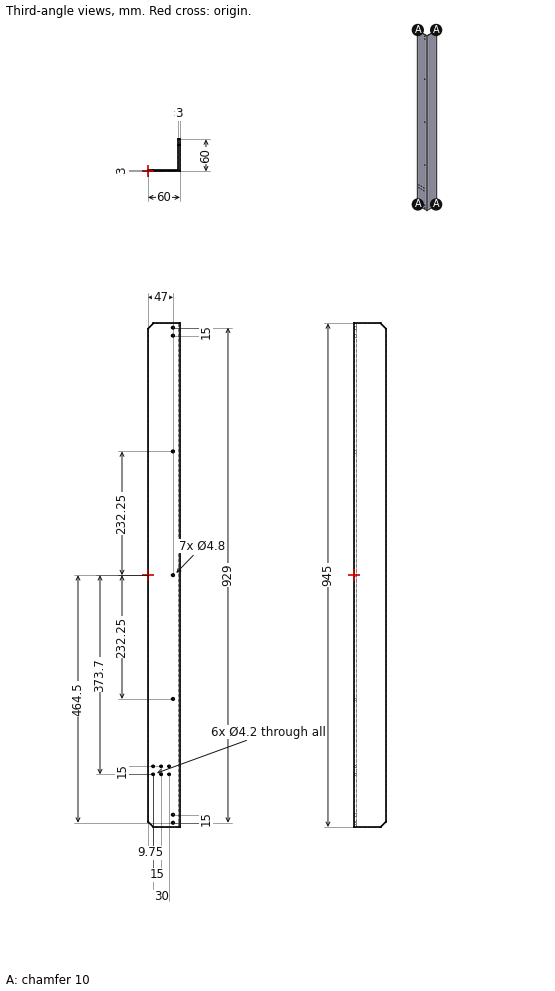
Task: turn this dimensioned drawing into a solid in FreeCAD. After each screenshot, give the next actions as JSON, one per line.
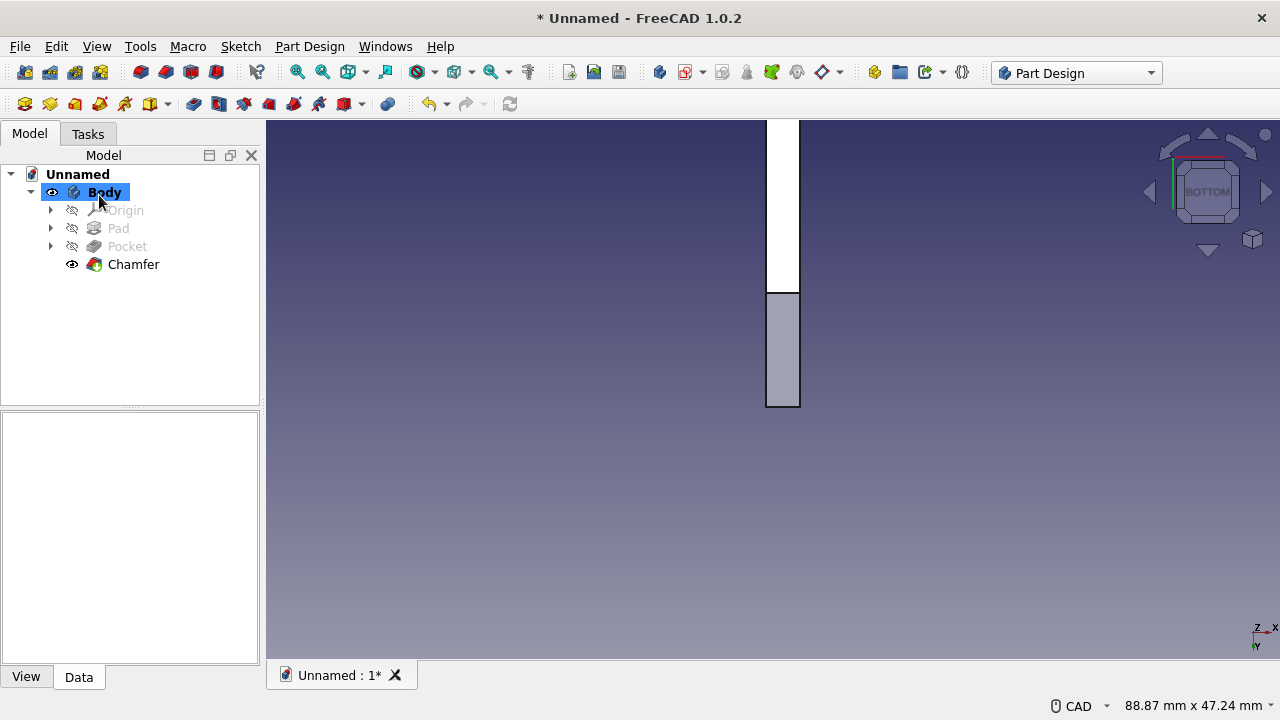
{"action": "left_click", "coordinate": [298, 72]}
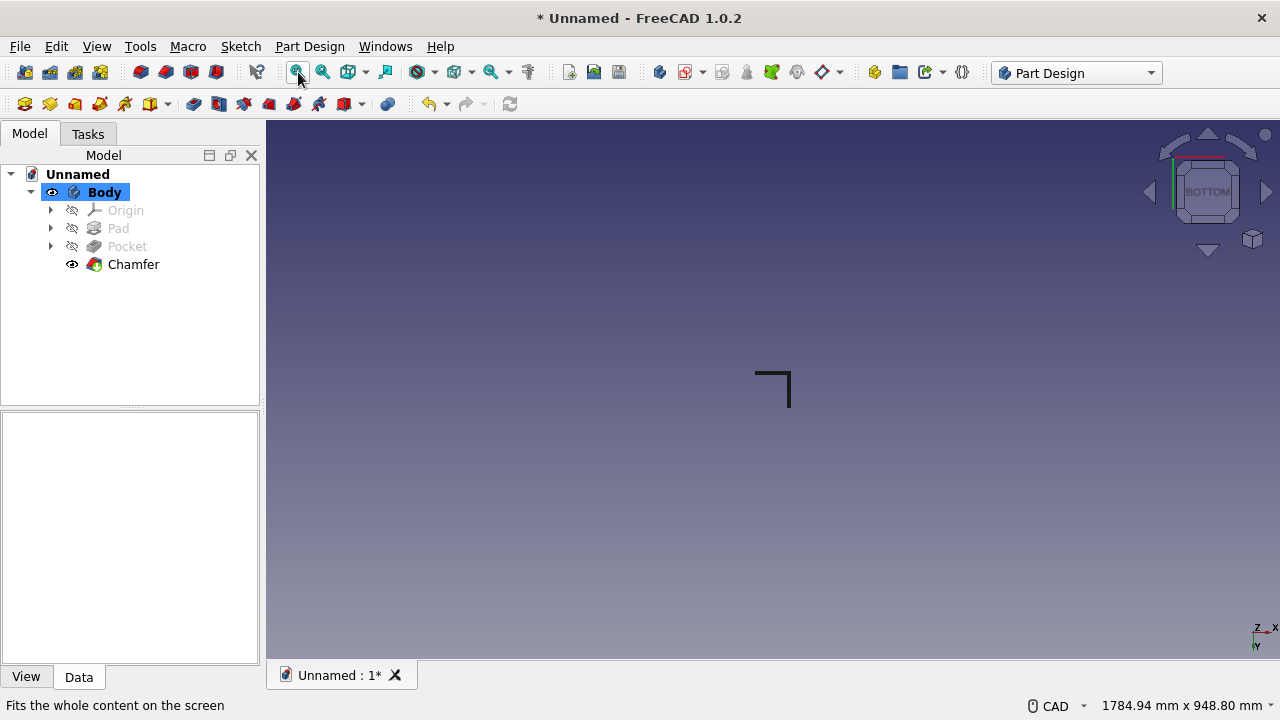
{"action": "key", "text": "4"}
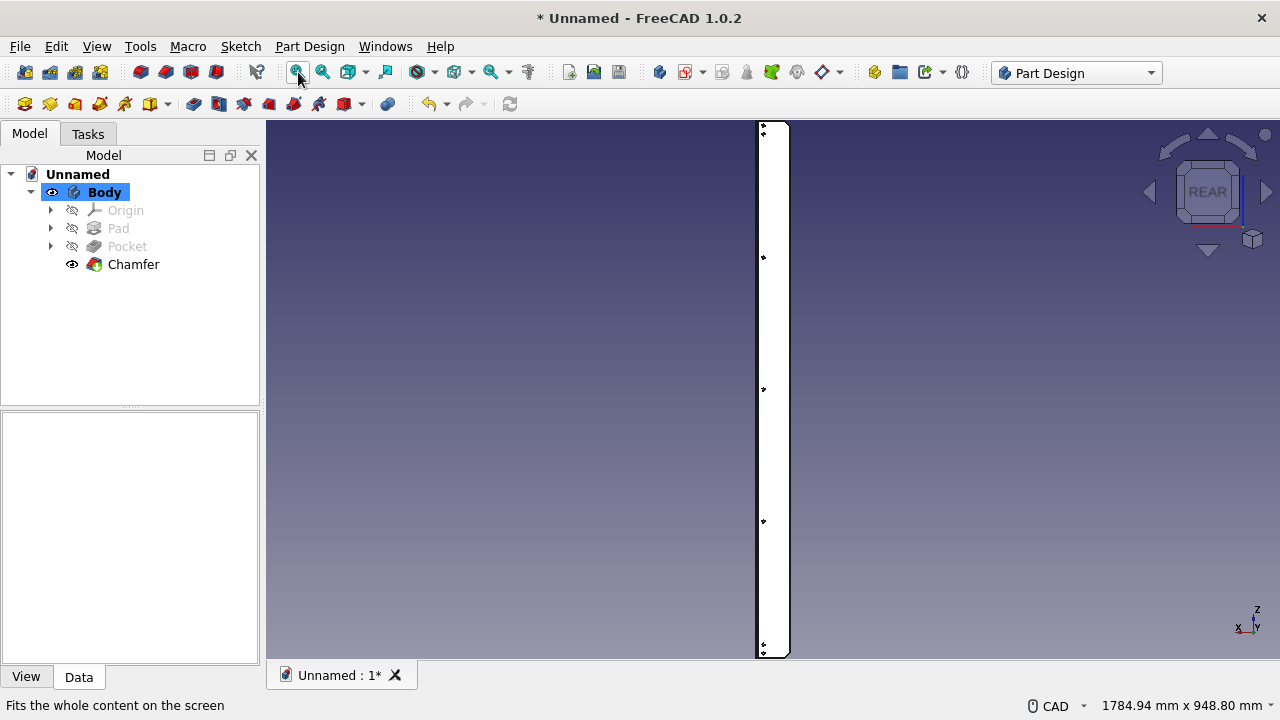
{"action": "left_click", "coordinate": [774, 158]}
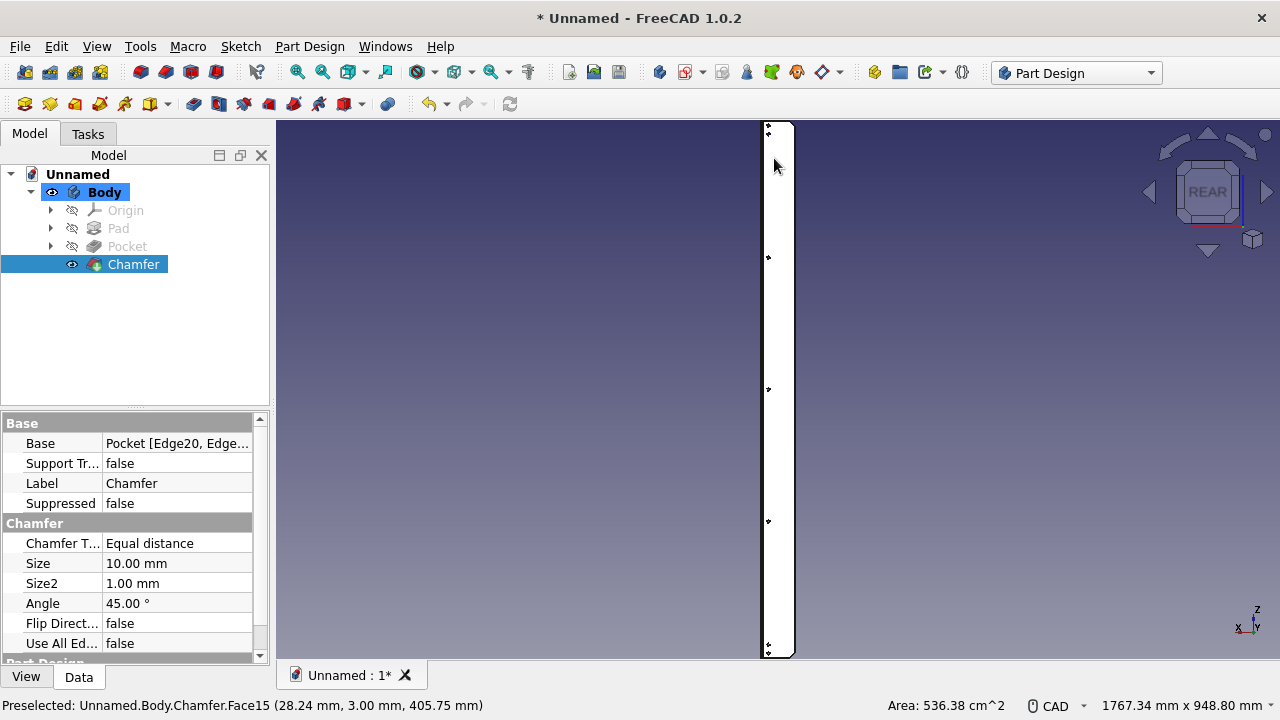
{"action": "left_click", "coordinate": [684, 72]}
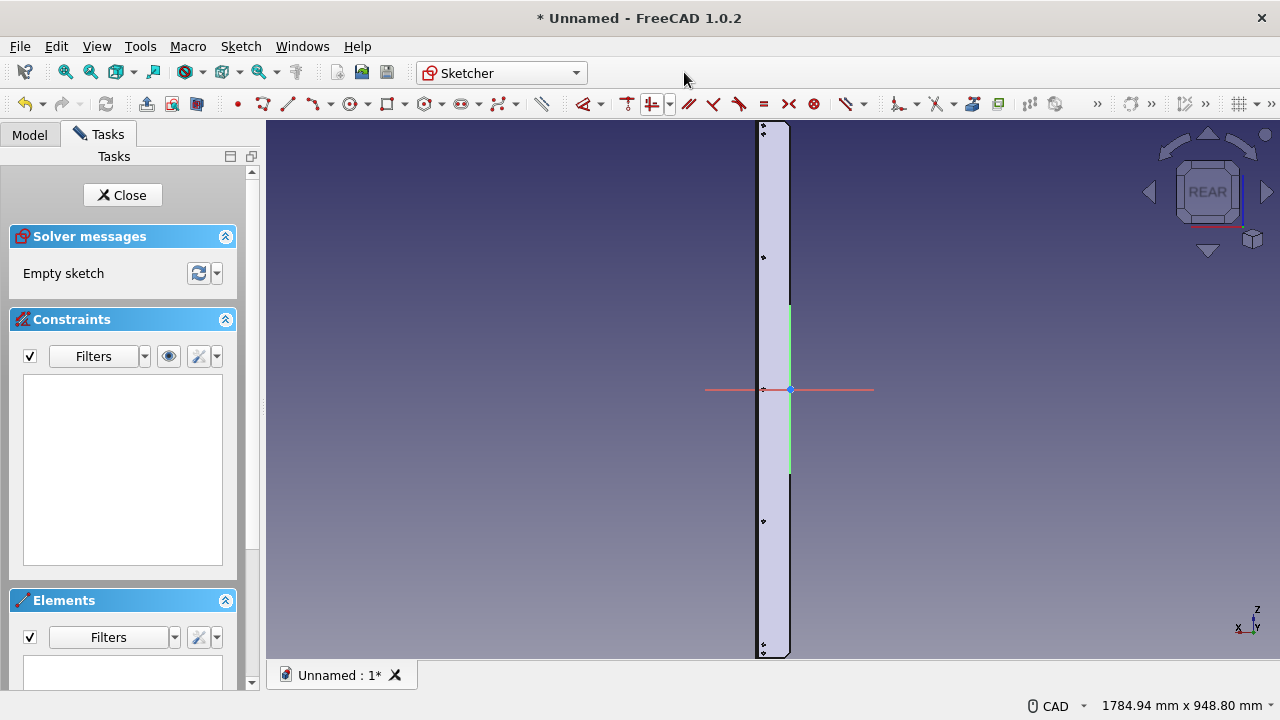
{"action": "left_click", "coordinate": [197, 104]}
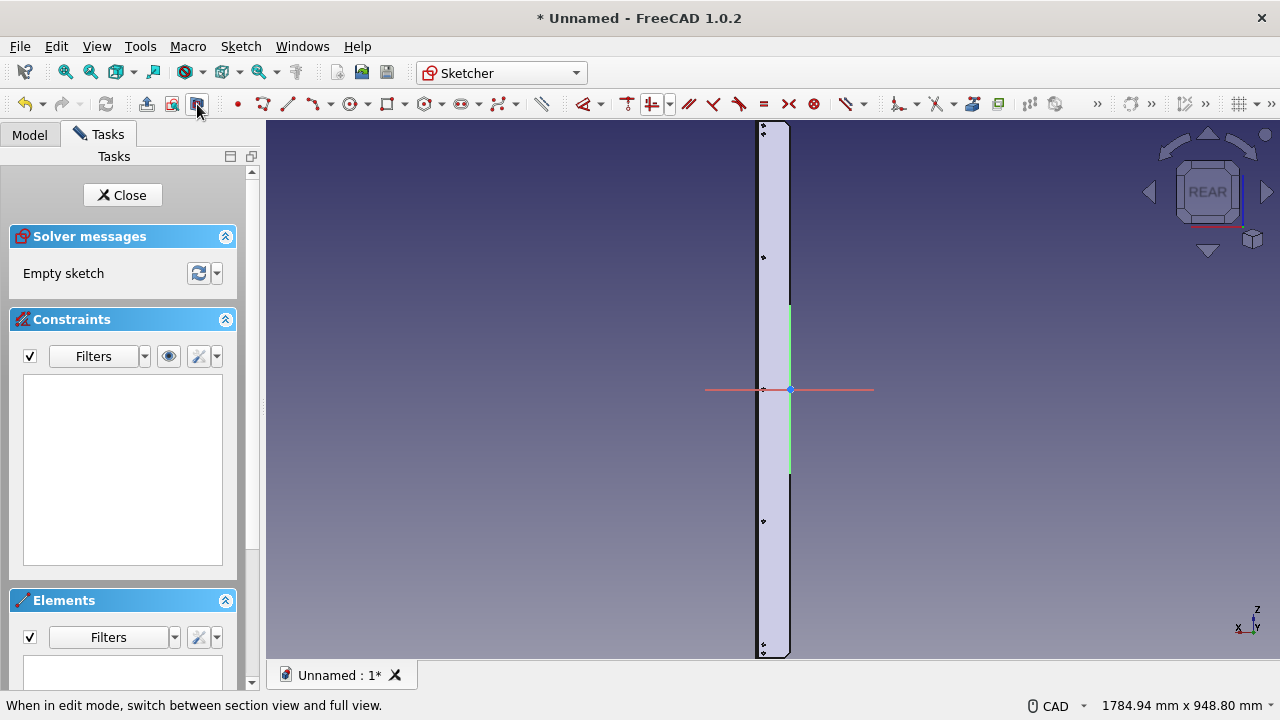
{"action": "scroll", "coordinate": [780, 608], "scroll_direction": "up", "scroll_amount": 15}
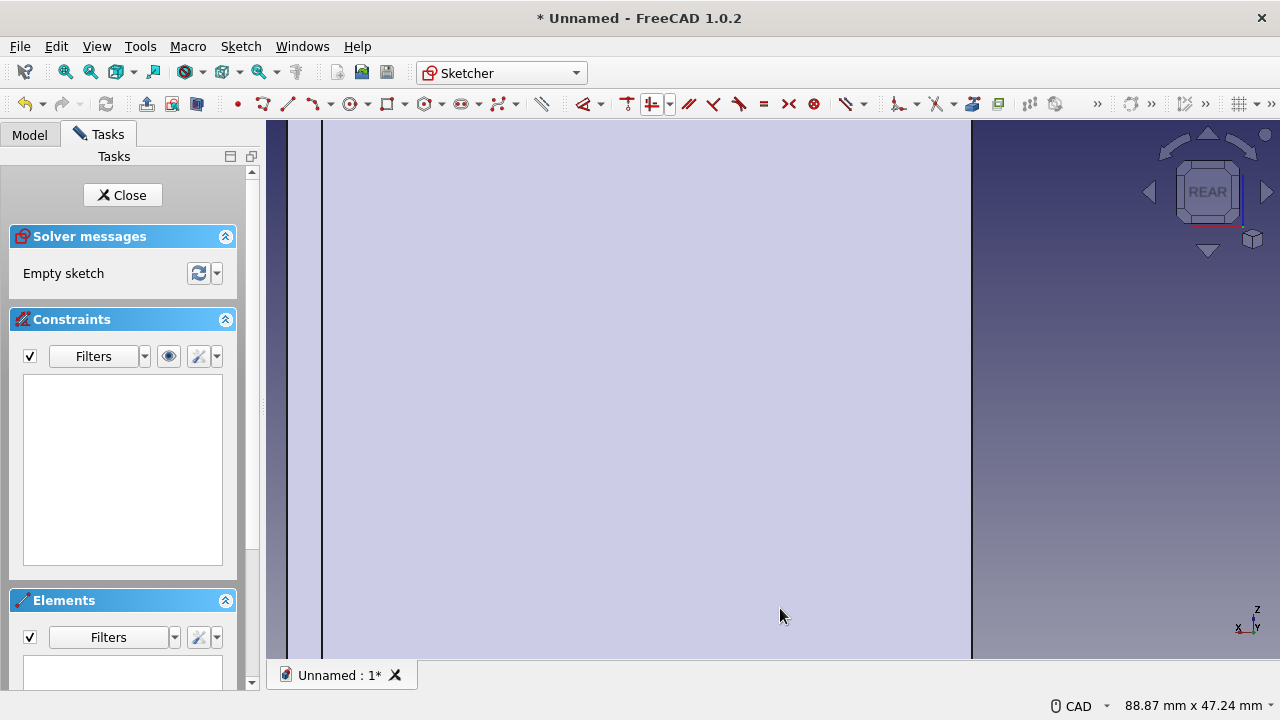
{"action": "scroll", "coordinate": [659, 362], "scroll_direction": "up", "scroll_amount": 2}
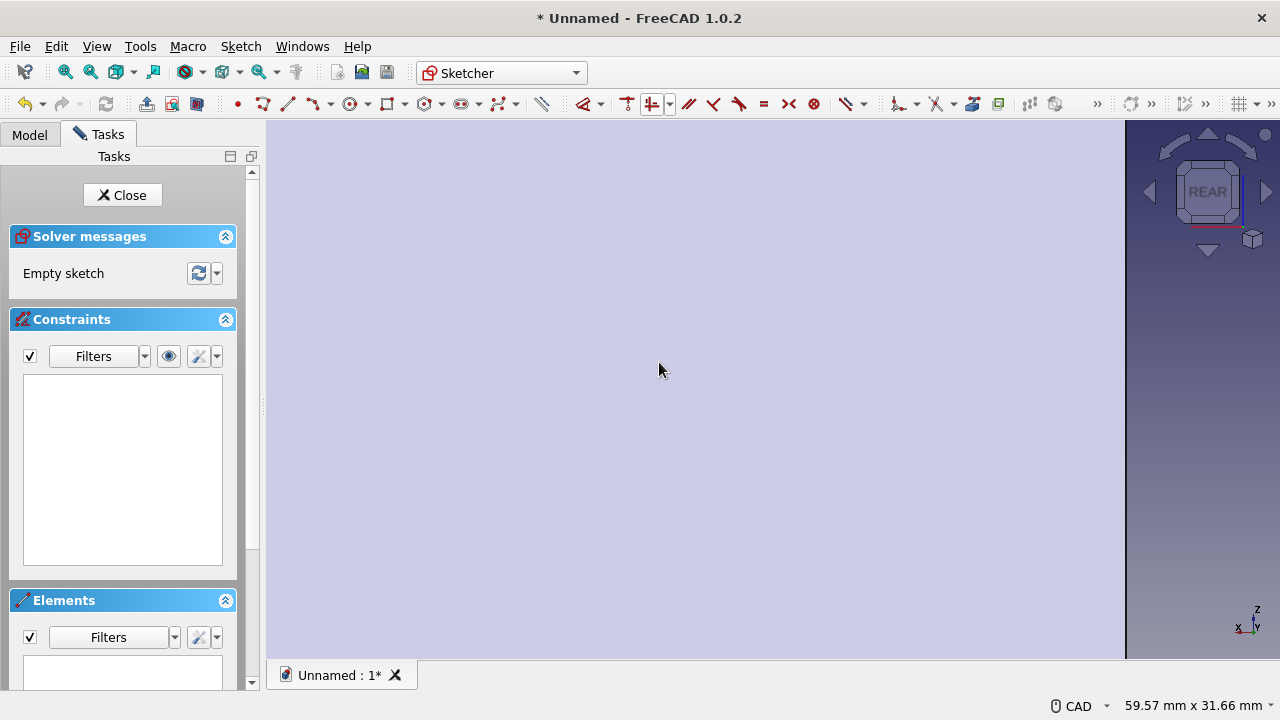
{"action": "left_click", "coordinate": [350, 104]}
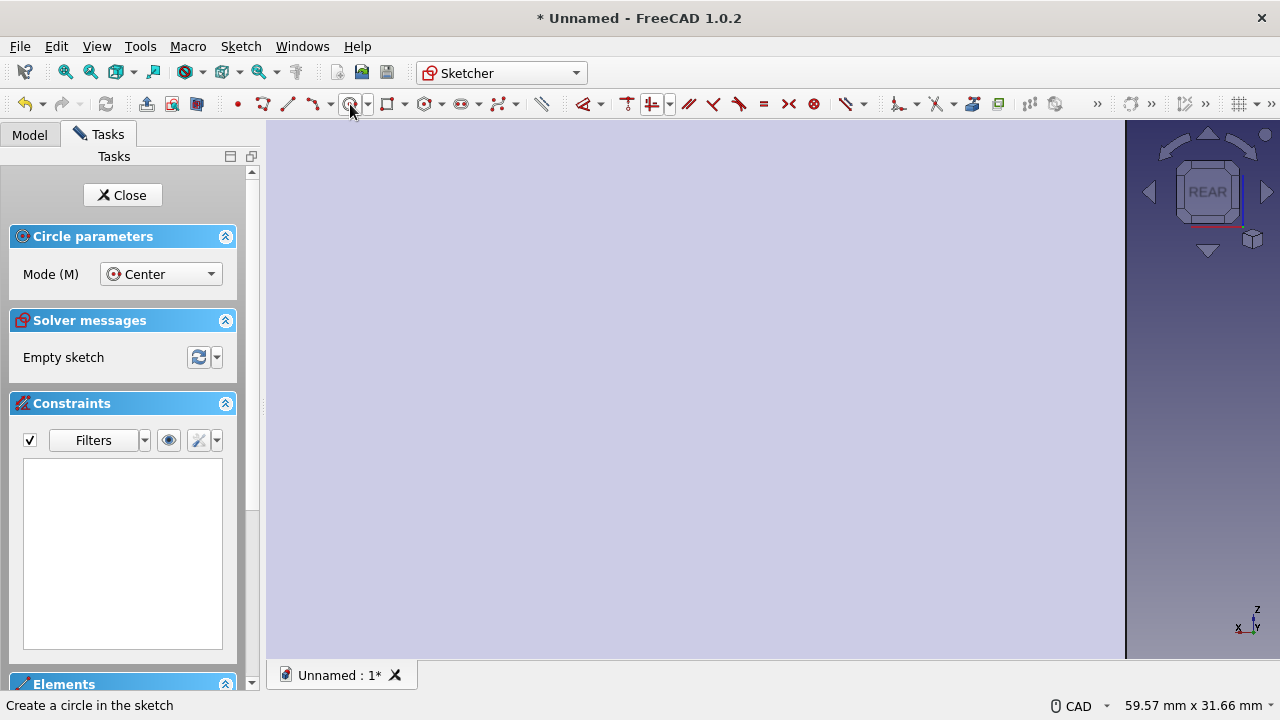
{"action": "left_click", "coordinate": [960, 517]}
{"action": "left_click", "coordinate": [985, 492]}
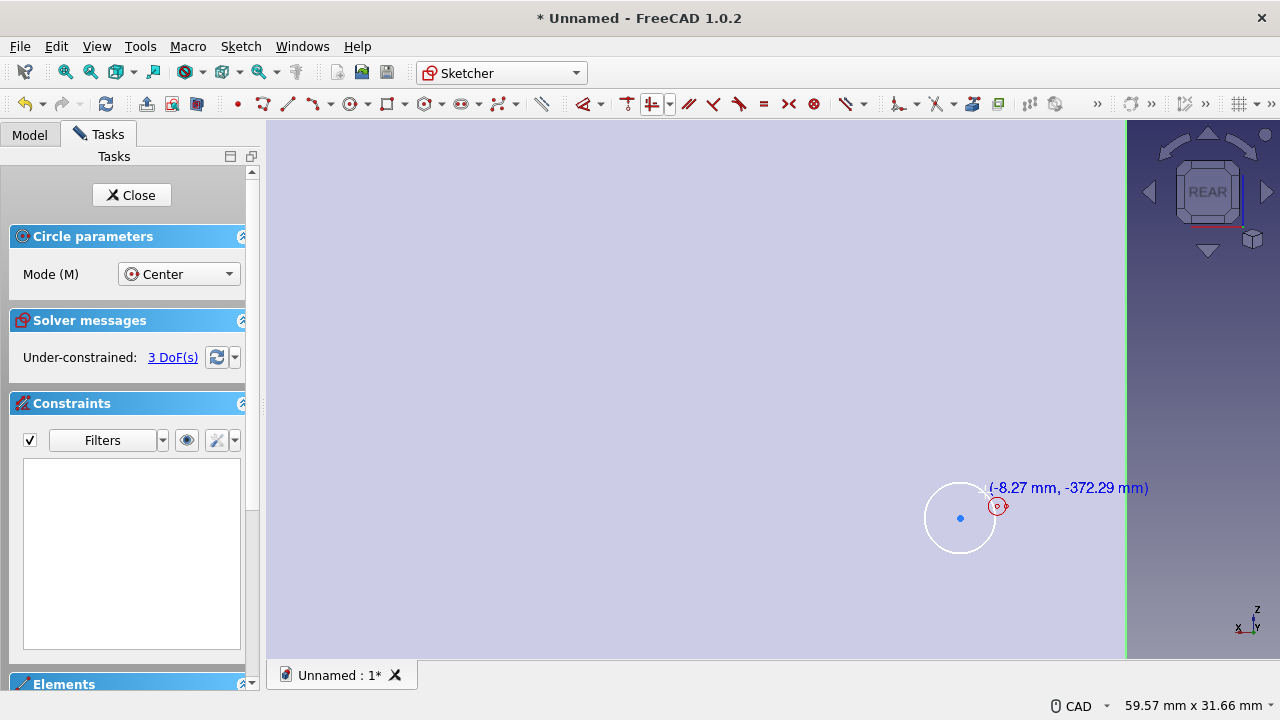
{"action": "left_click", "coordinate": [449, 517]}
{"action": "left_click", "coordinate": [474, 492]}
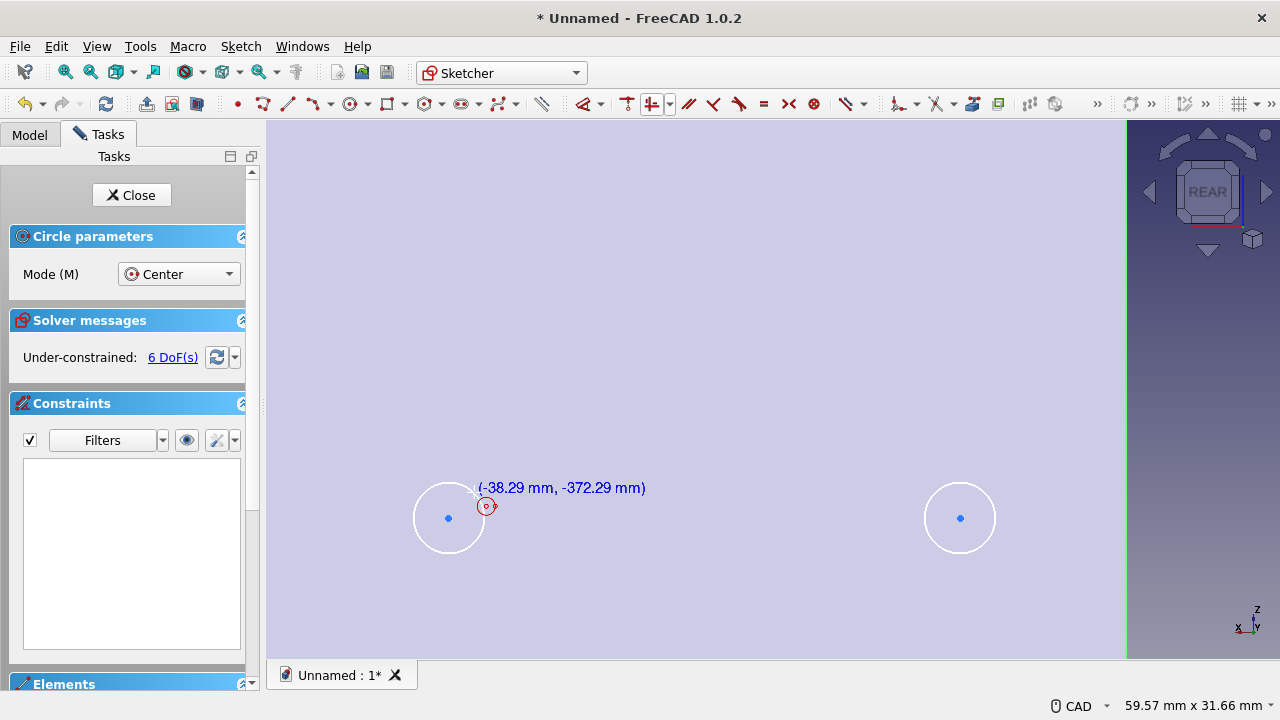
{"action": "left_click", "coordinate": [704, 262]}
{"action": "left_click", "coordinate": [730, 236]}